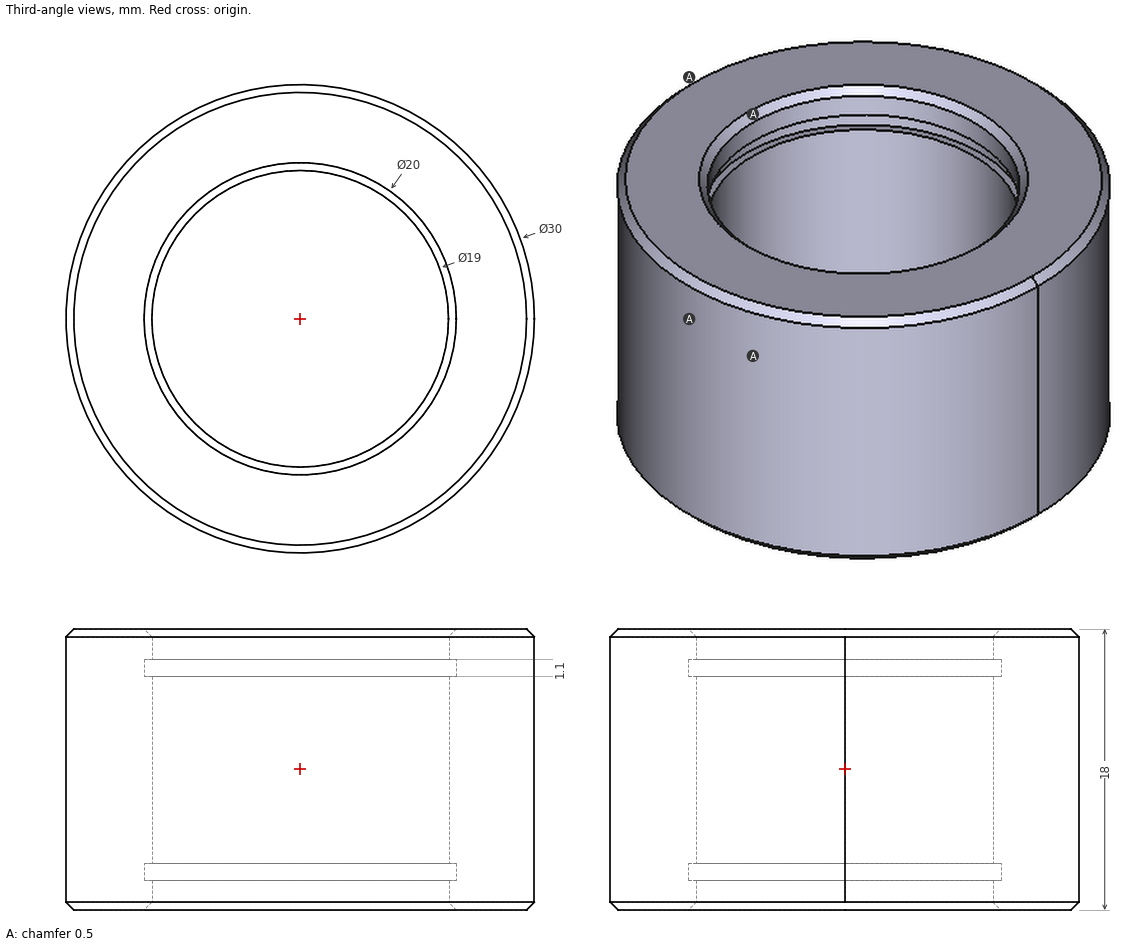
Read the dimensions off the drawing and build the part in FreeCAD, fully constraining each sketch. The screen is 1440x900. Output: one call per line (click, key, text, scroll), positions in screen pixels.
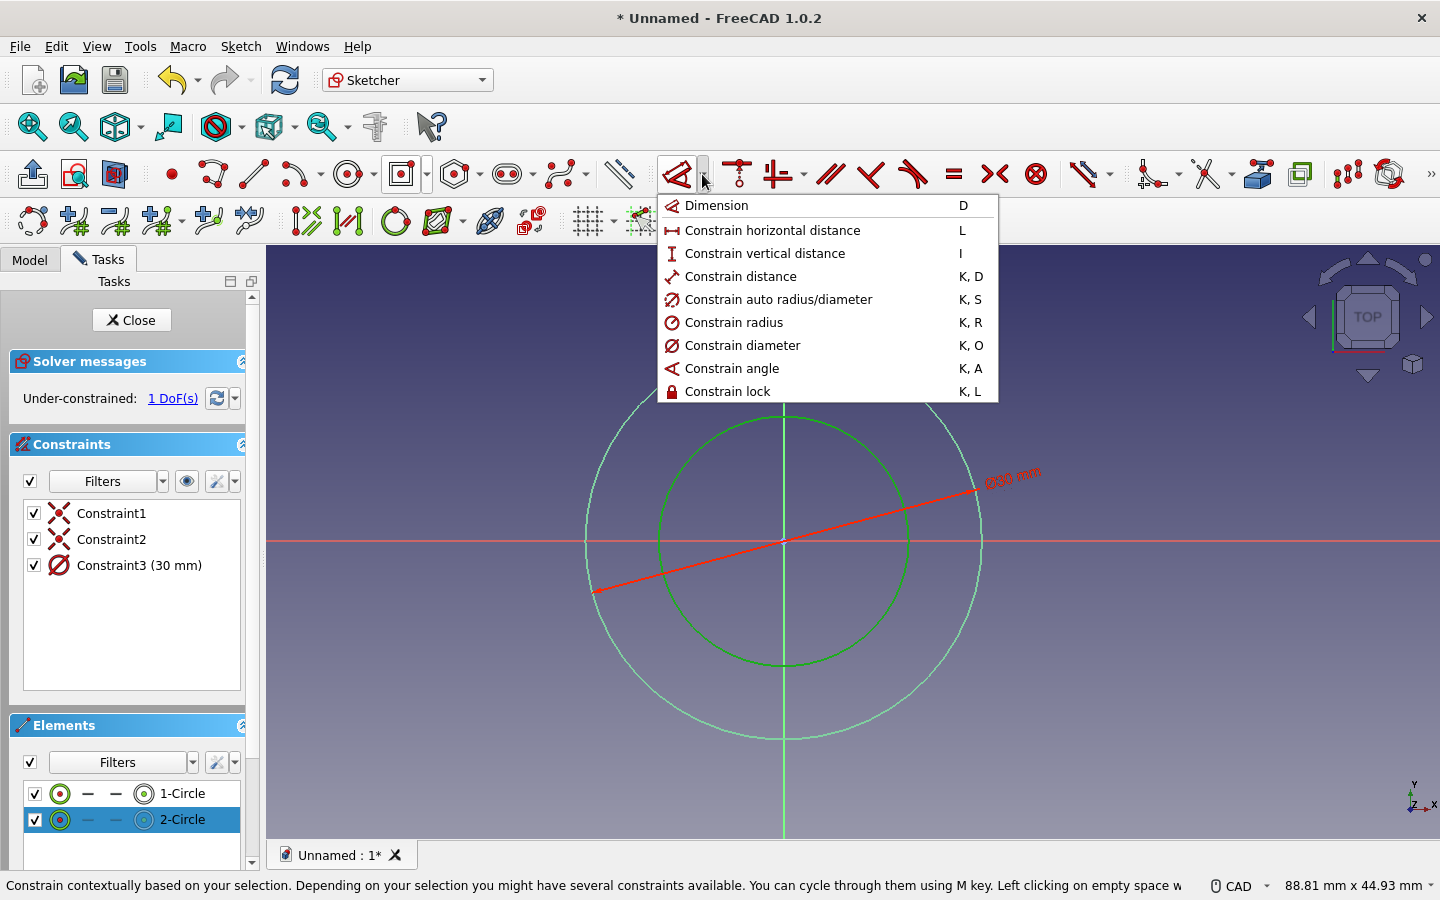
click(828, 346)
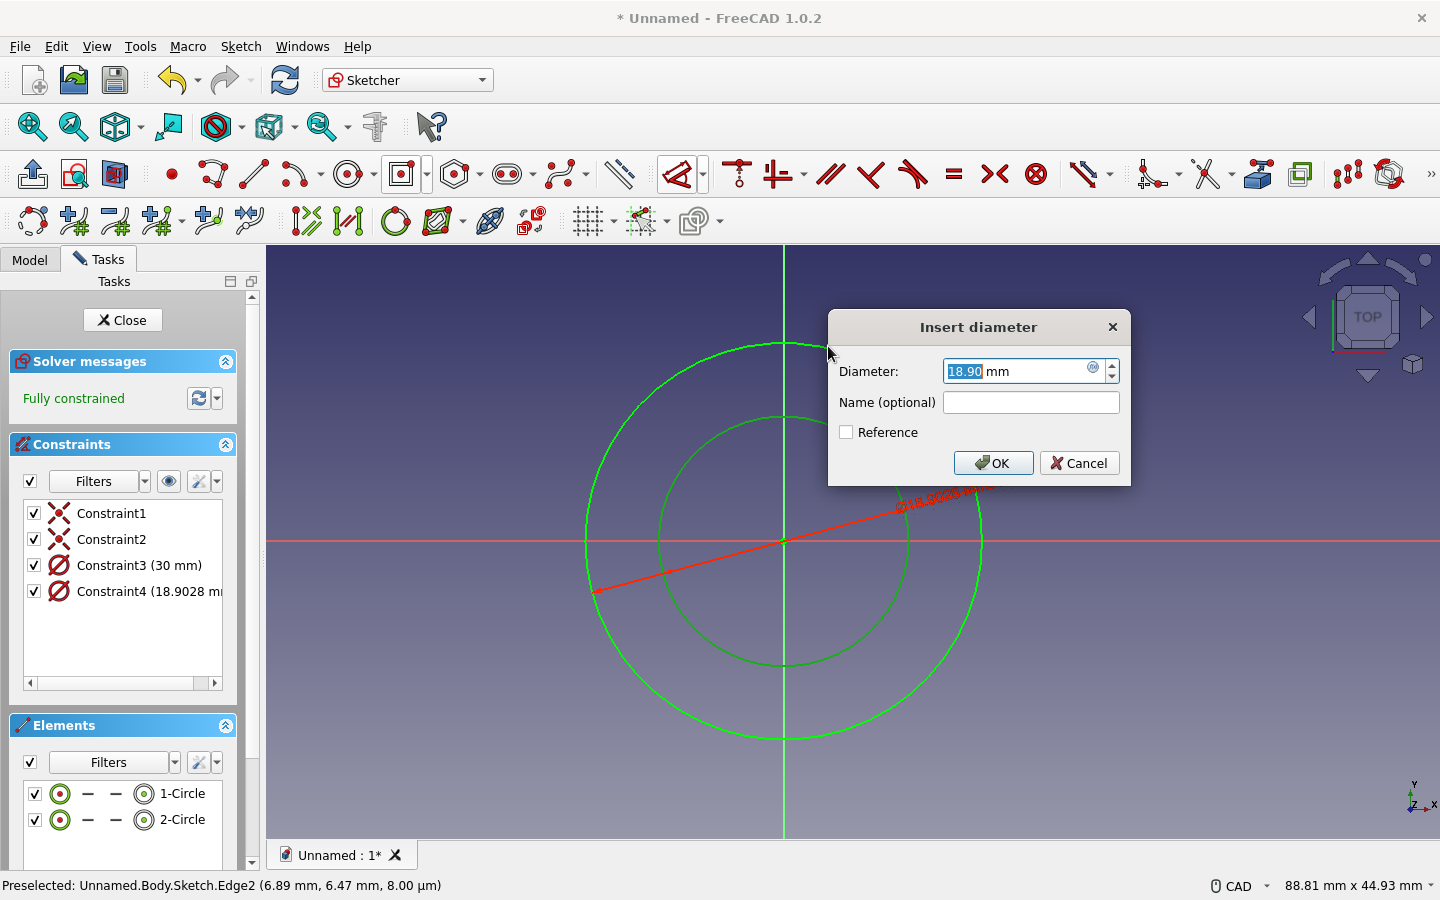
text(19)
key(Return)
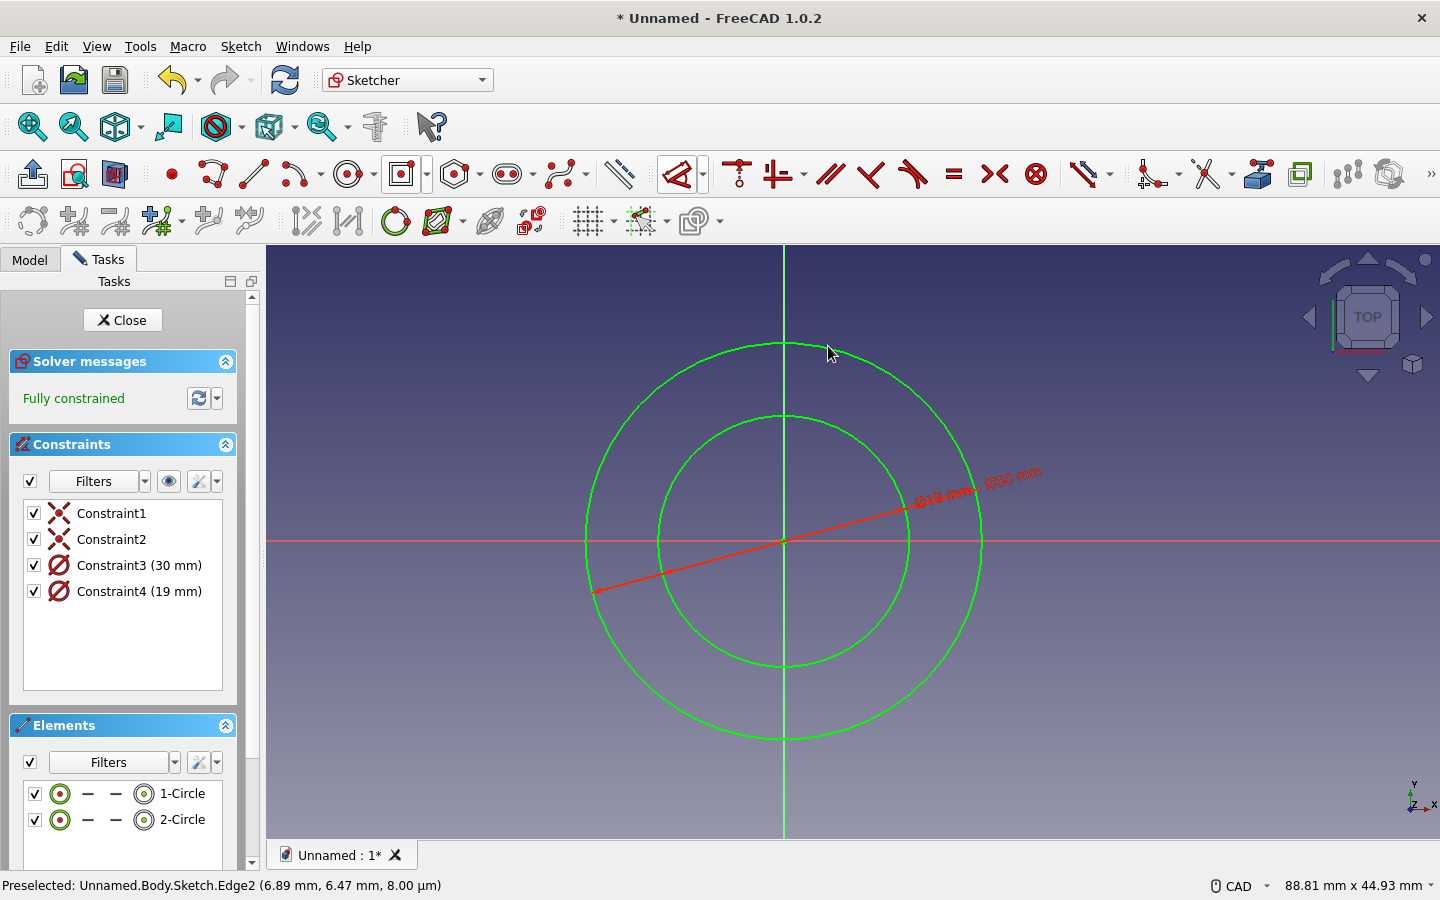
click(123, 320)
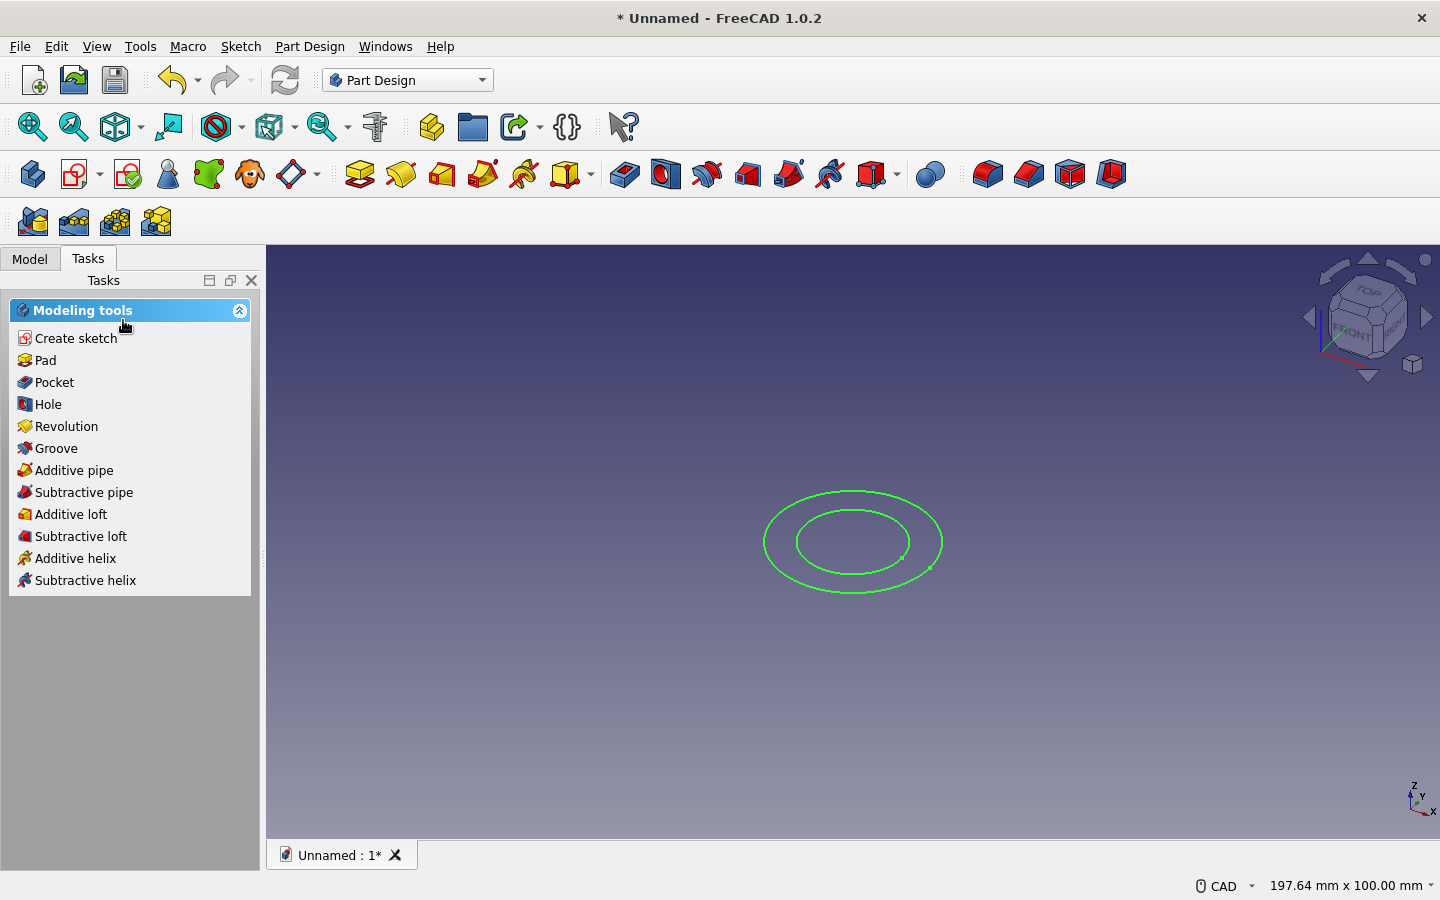
click(360, 174)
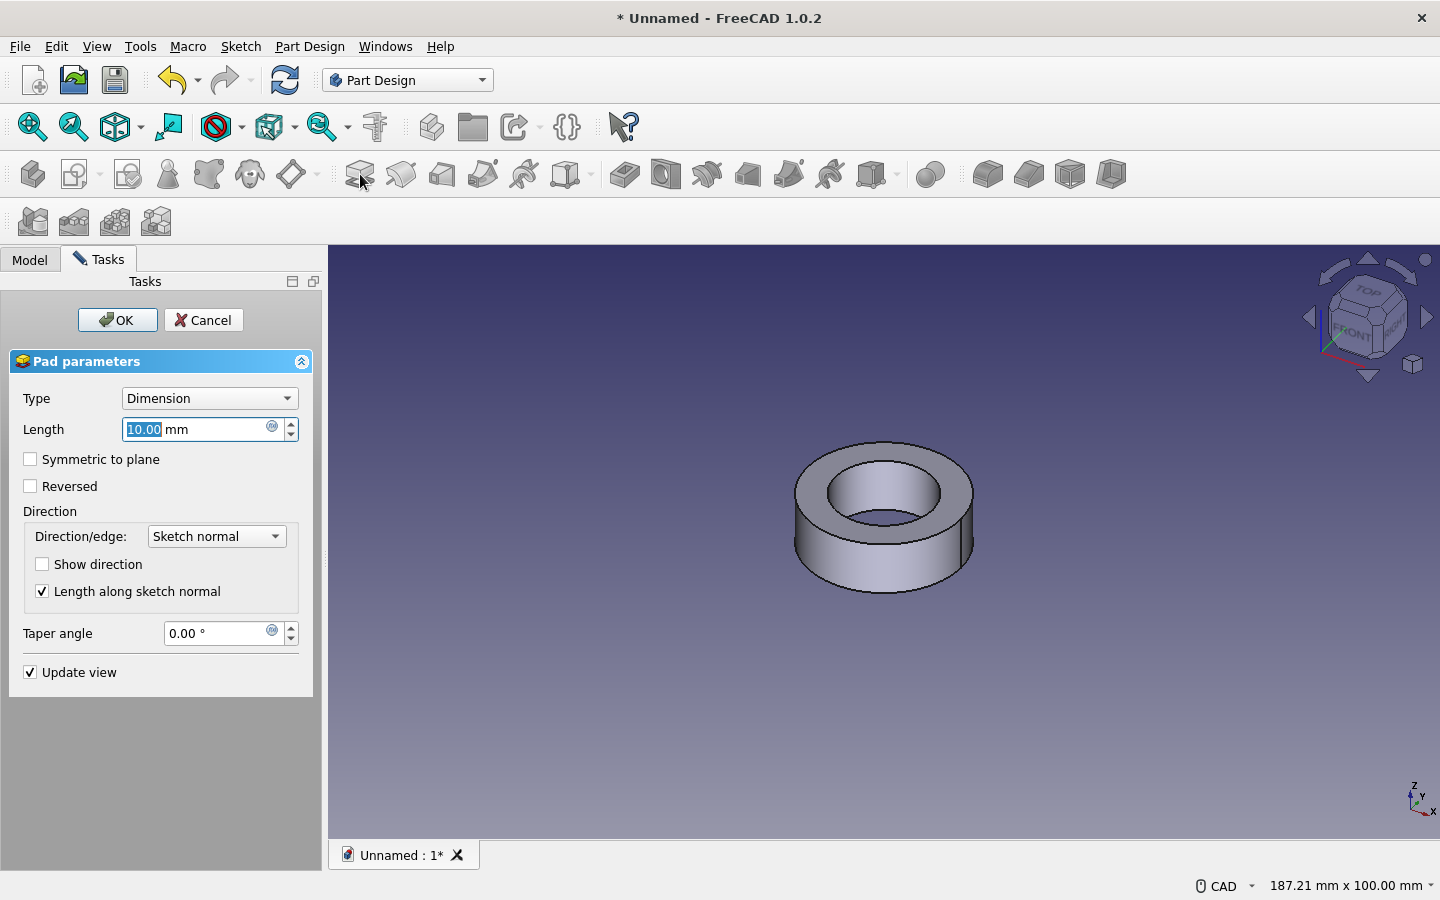
text(18)
key(Tab)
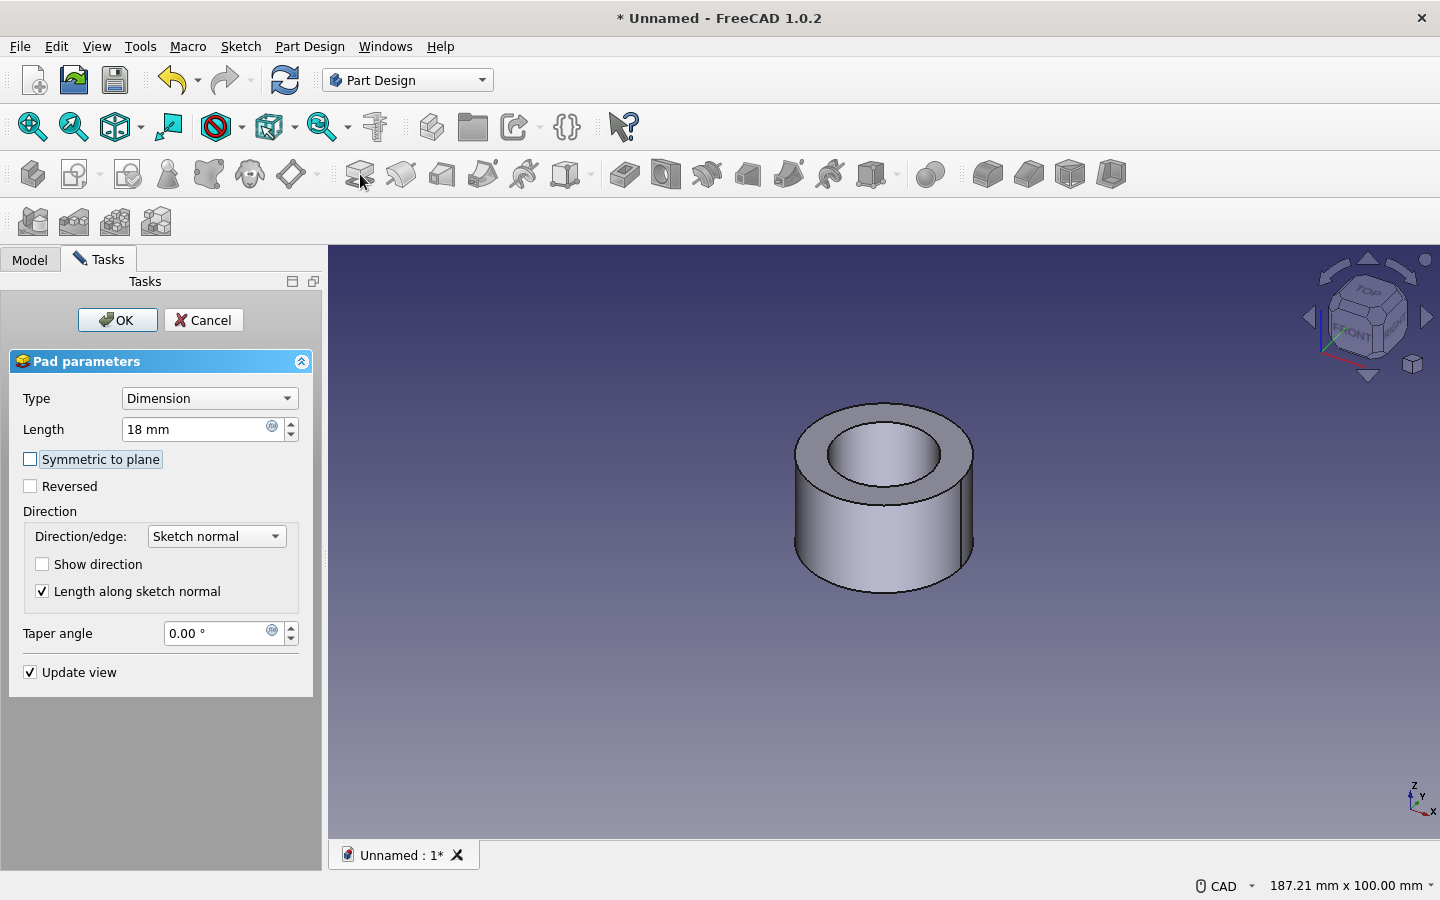
click(31, 459)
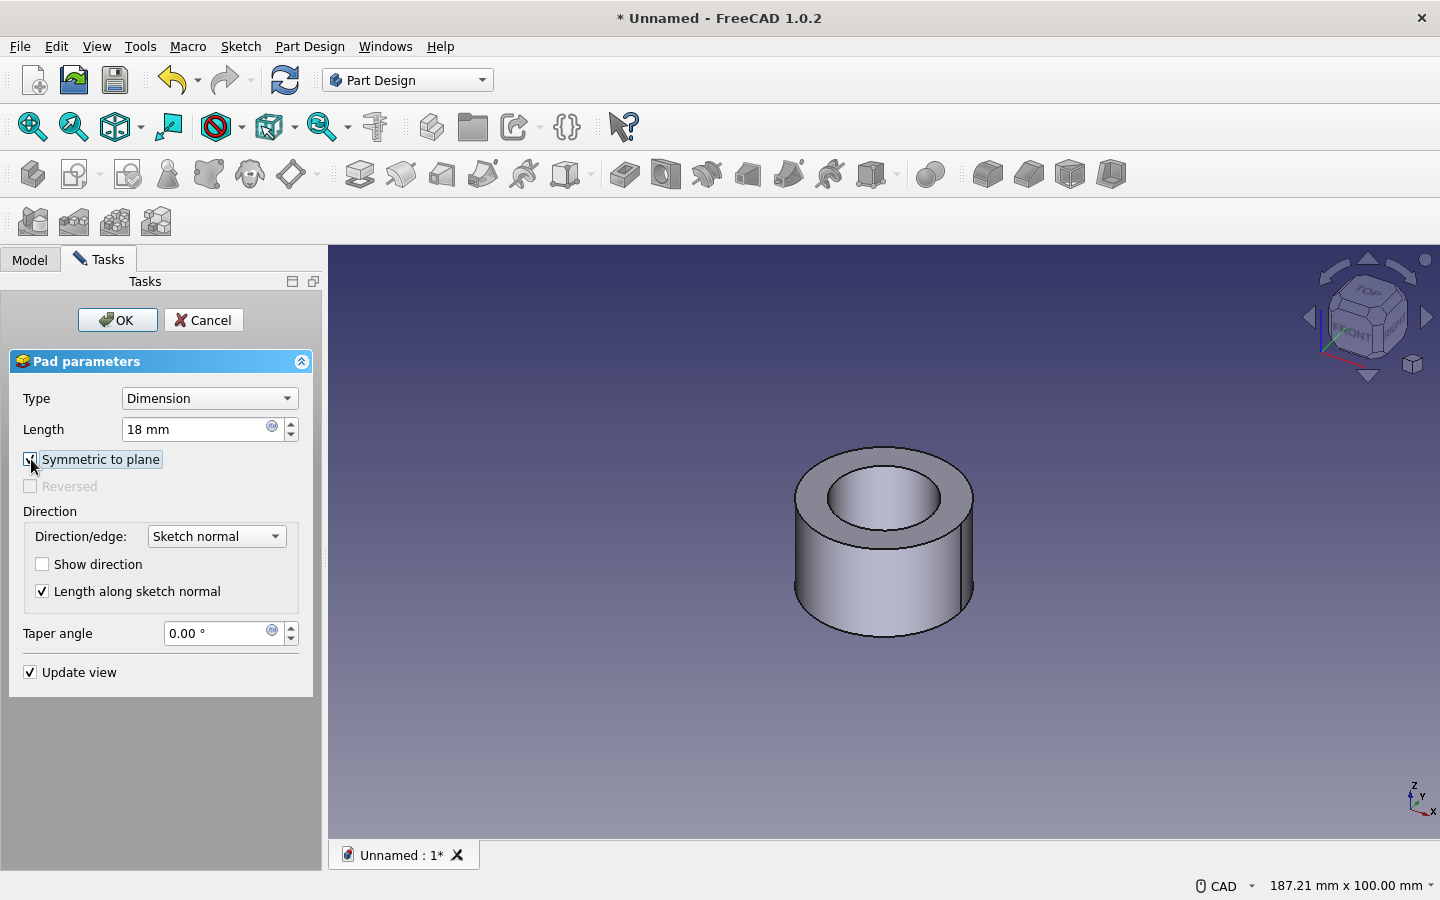
click(118, 320)